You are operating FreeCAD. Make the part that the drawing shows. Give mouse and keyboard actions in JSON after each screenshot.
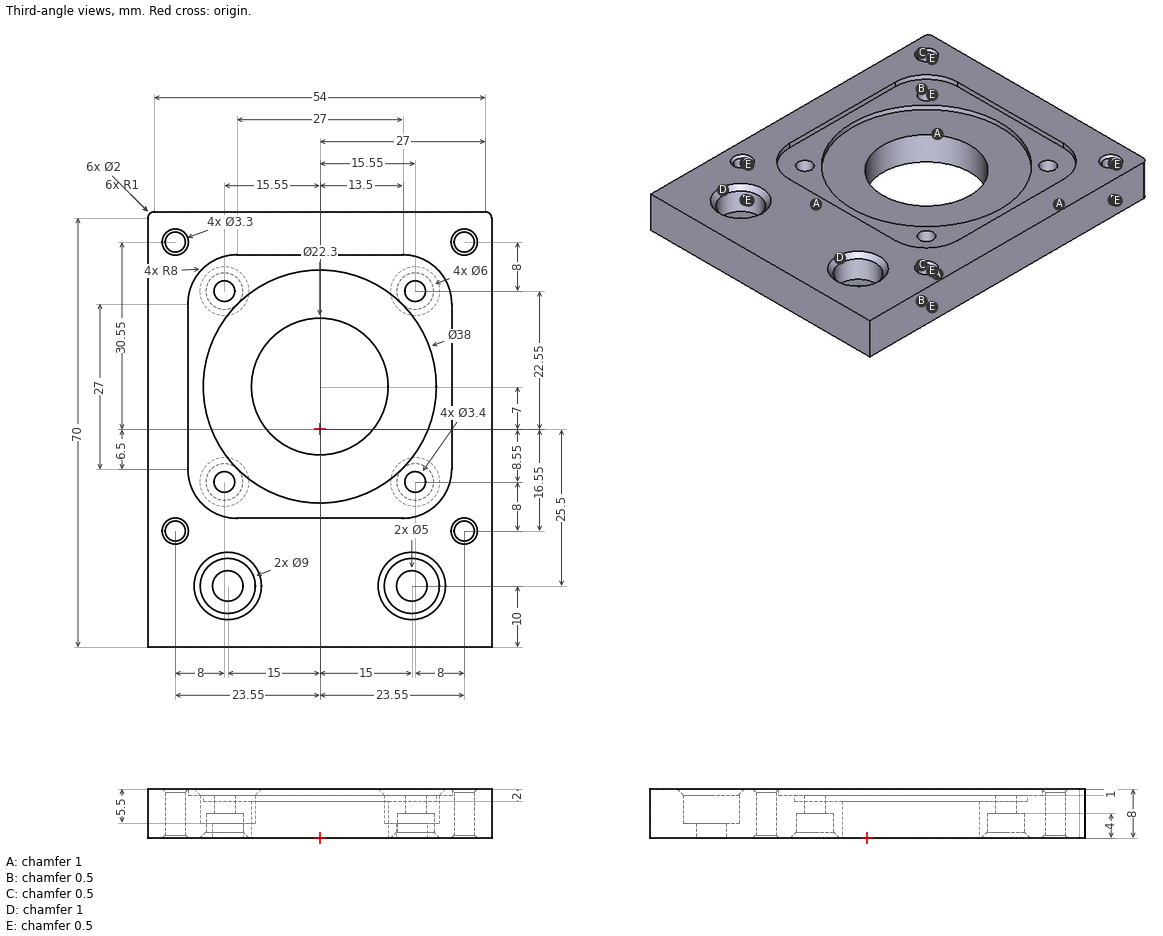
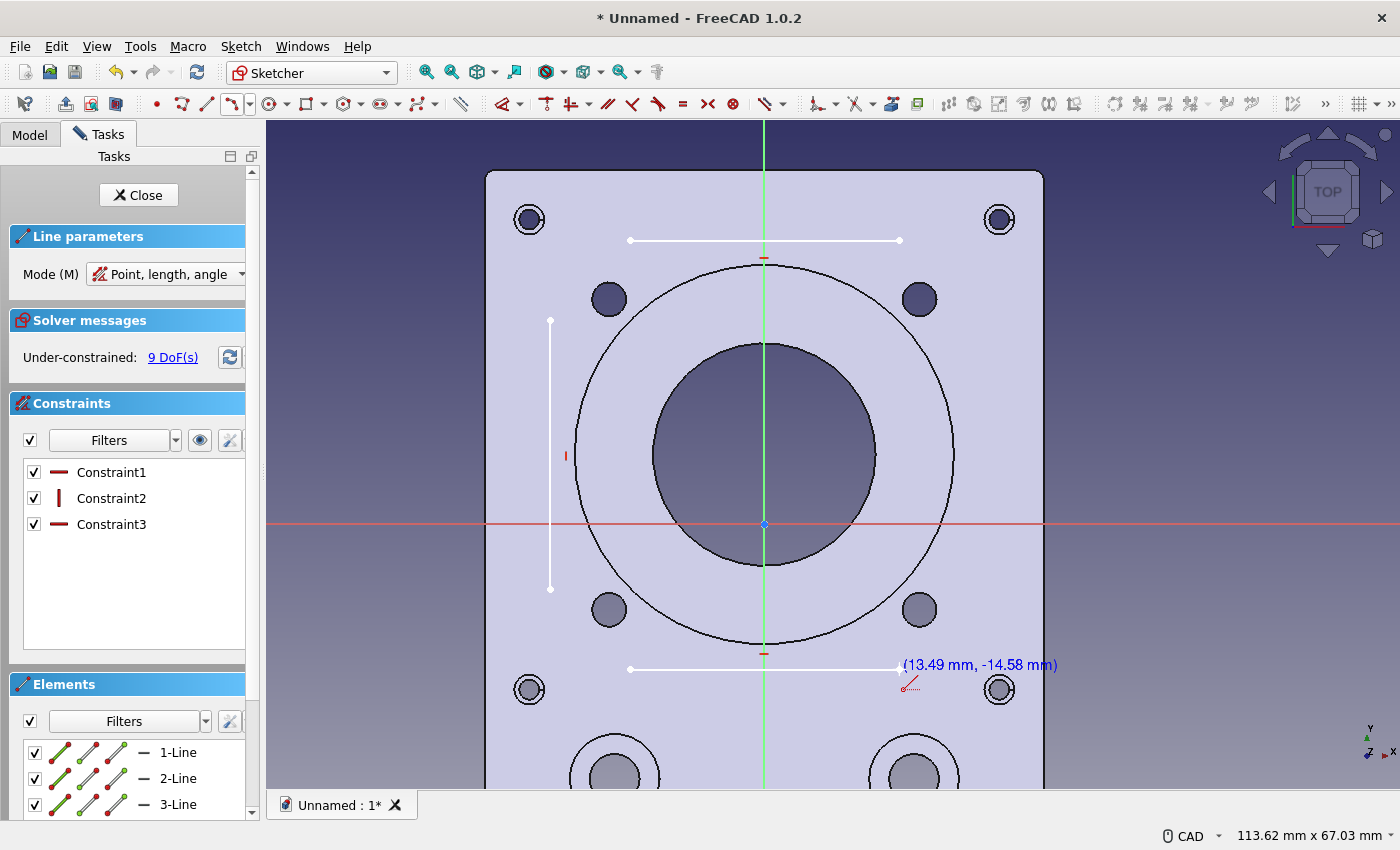
{"action": "left_click", "coordinate": [979, 589]}
{"action": "left_click", "coordinate": [979, 320]}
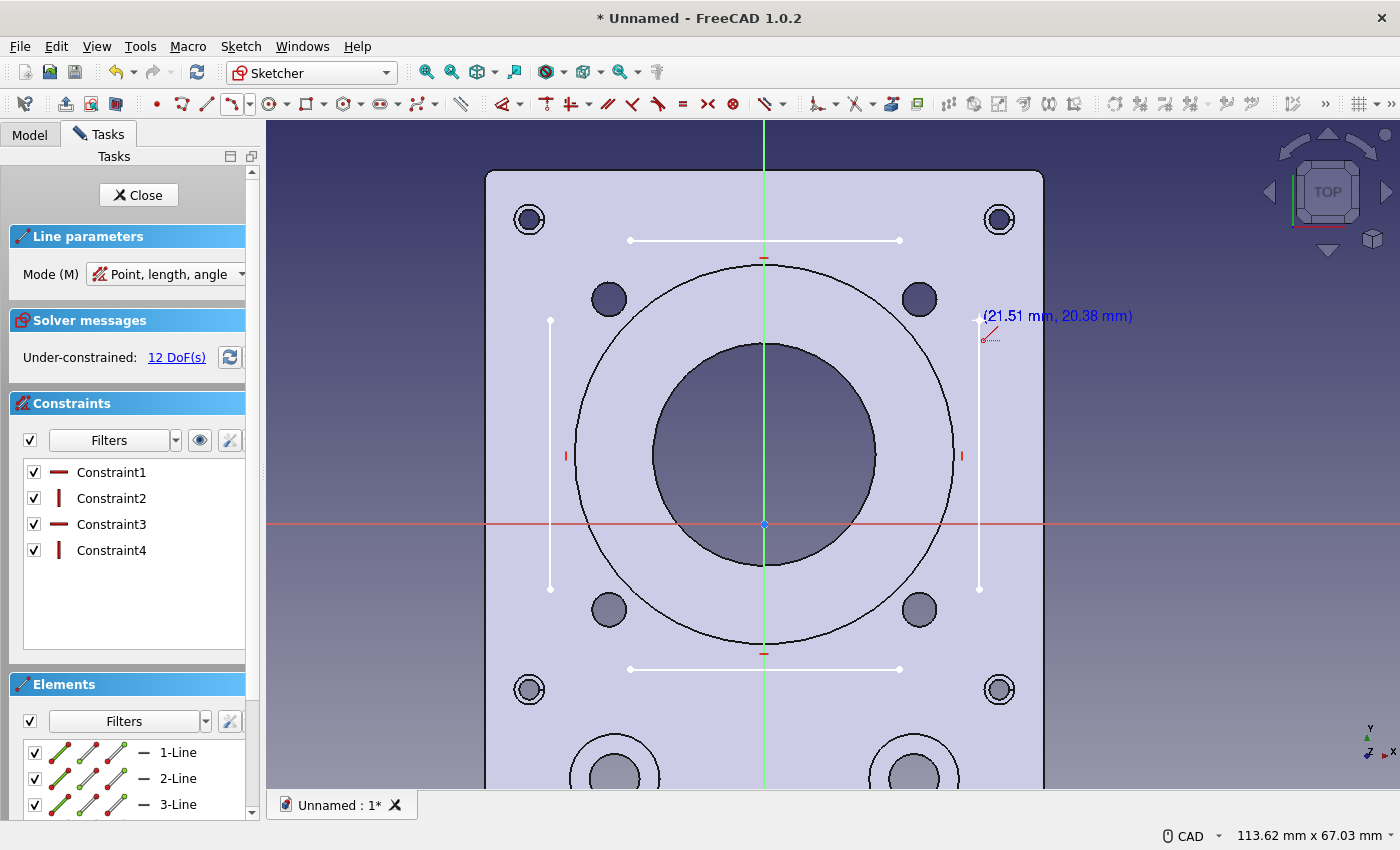
{"action": "key", "text": "g 3 a"}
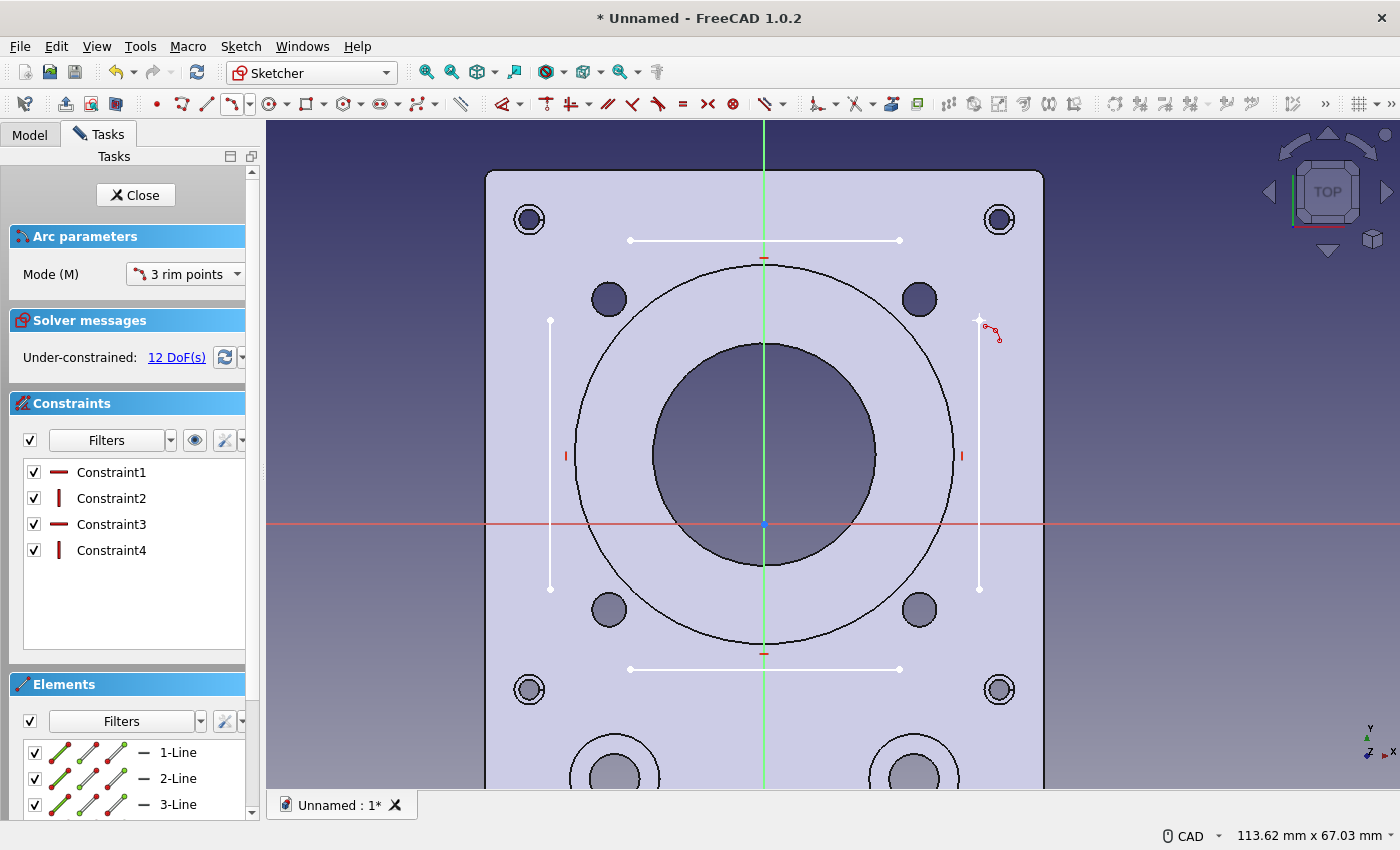
{"action": "left_click", "coordinate": [630, 241]}
{"action": "left_click", "coordinate": [550, 321]}
{"action": "left_click", "coordinate": [573, 263]}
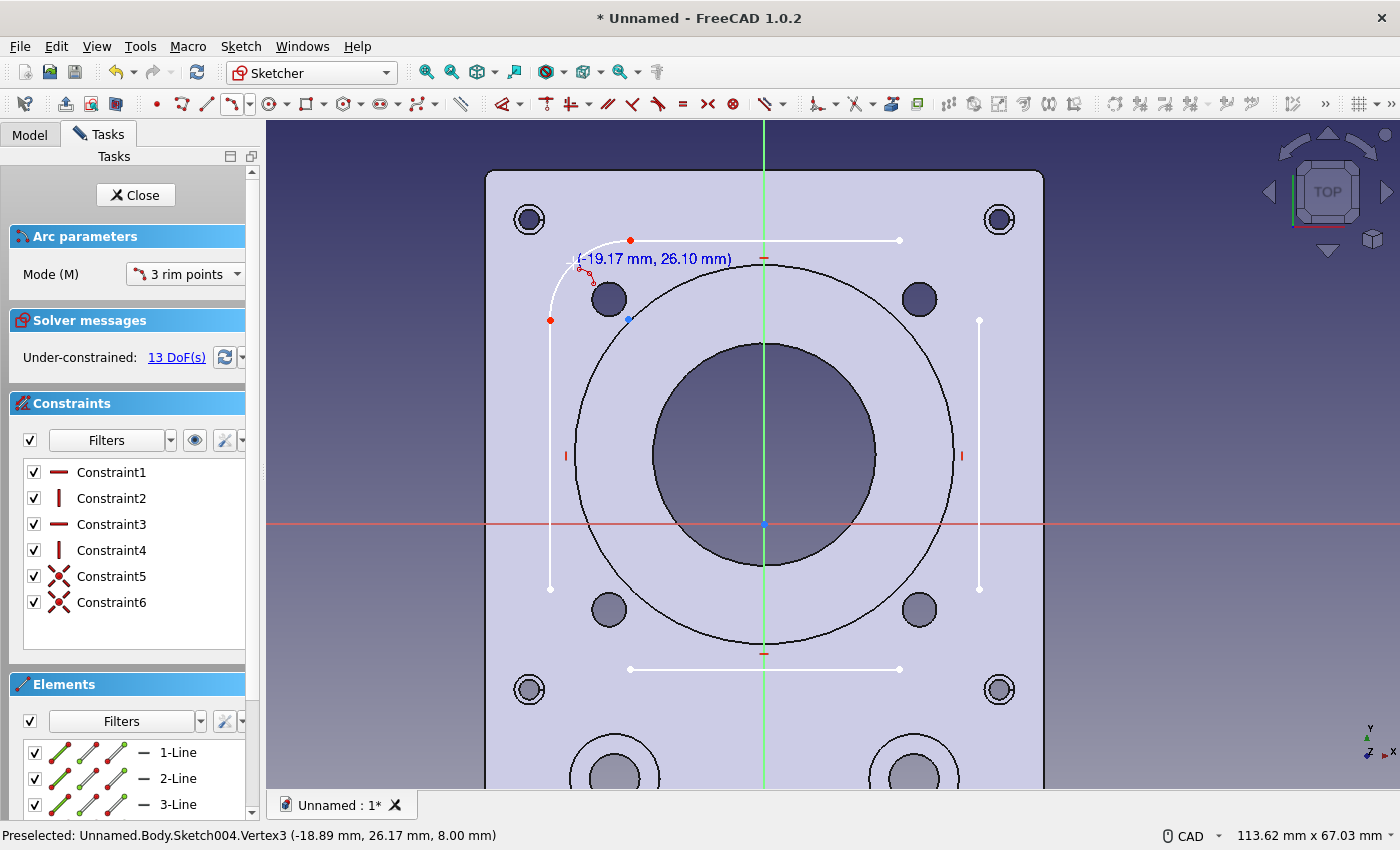
{"action": "left_click", "coordinate": [550, 590]}
{"action": "left_click", "coordinate": [630, 670]}
{"action": "left_click", "coordinate": [573, 646]}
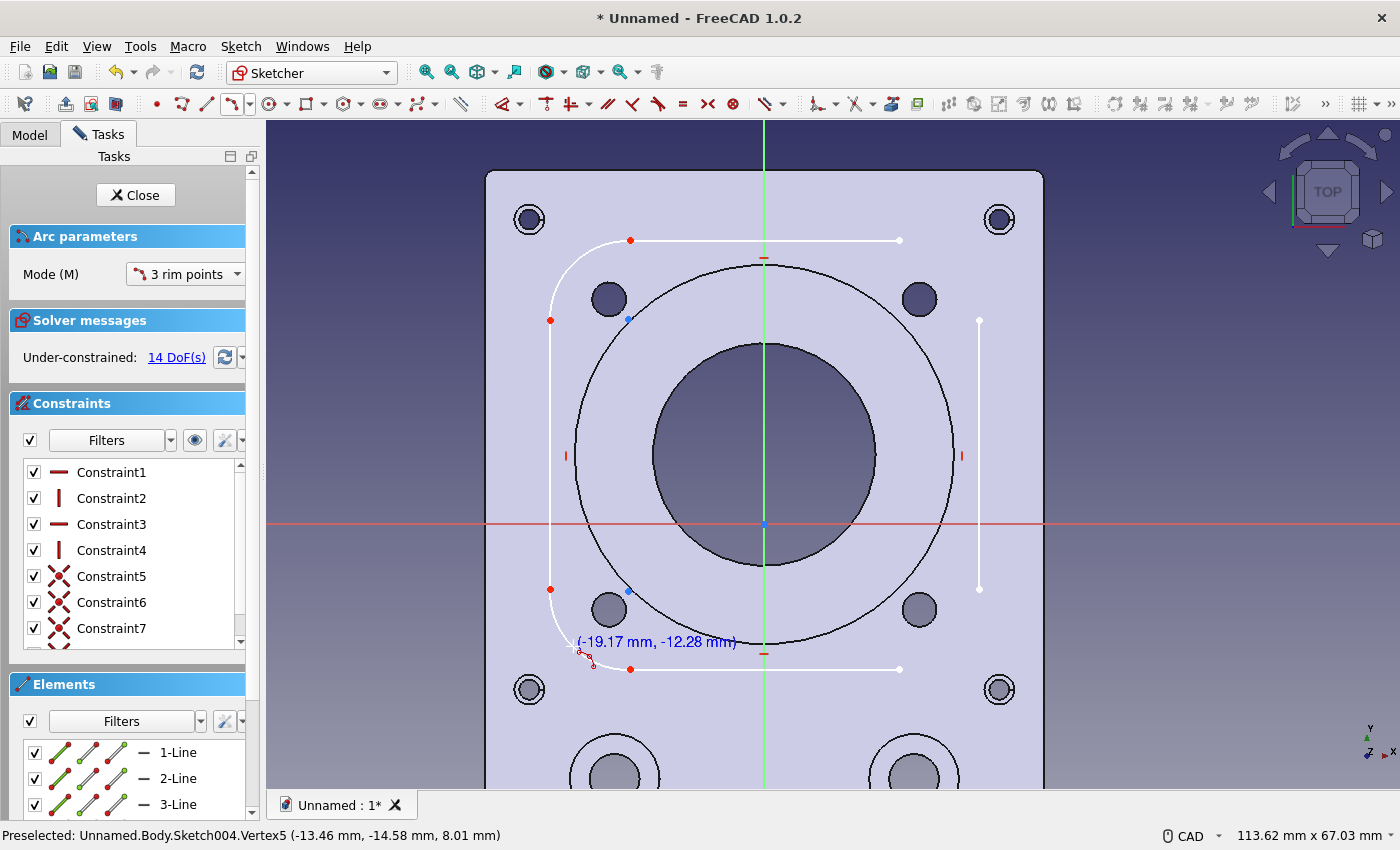
{"action": "left_click", "coordinate": [899, 670]}
{"action": "left_click", "coordinate": [979, 590]}
{"action": "left_click", "coordinate": [956, 646]}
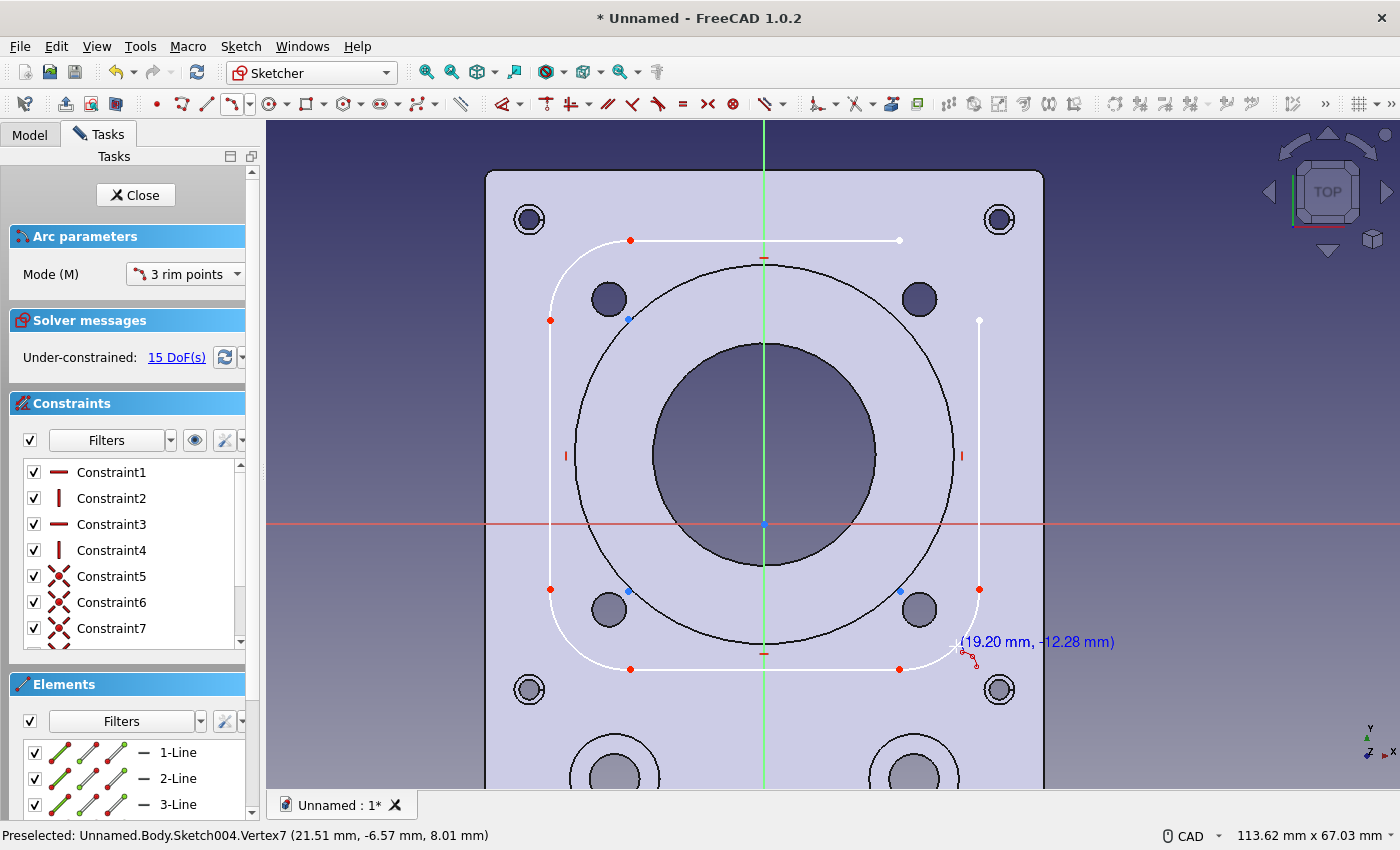
{"action": "left_click", "coordinate": [979, 321]}
{"action": "left_click", "coordinate": [899, 241]}
{"action": "left_click", "coordinate": [956, 263]}
{"action": "key", "text": "Escape"}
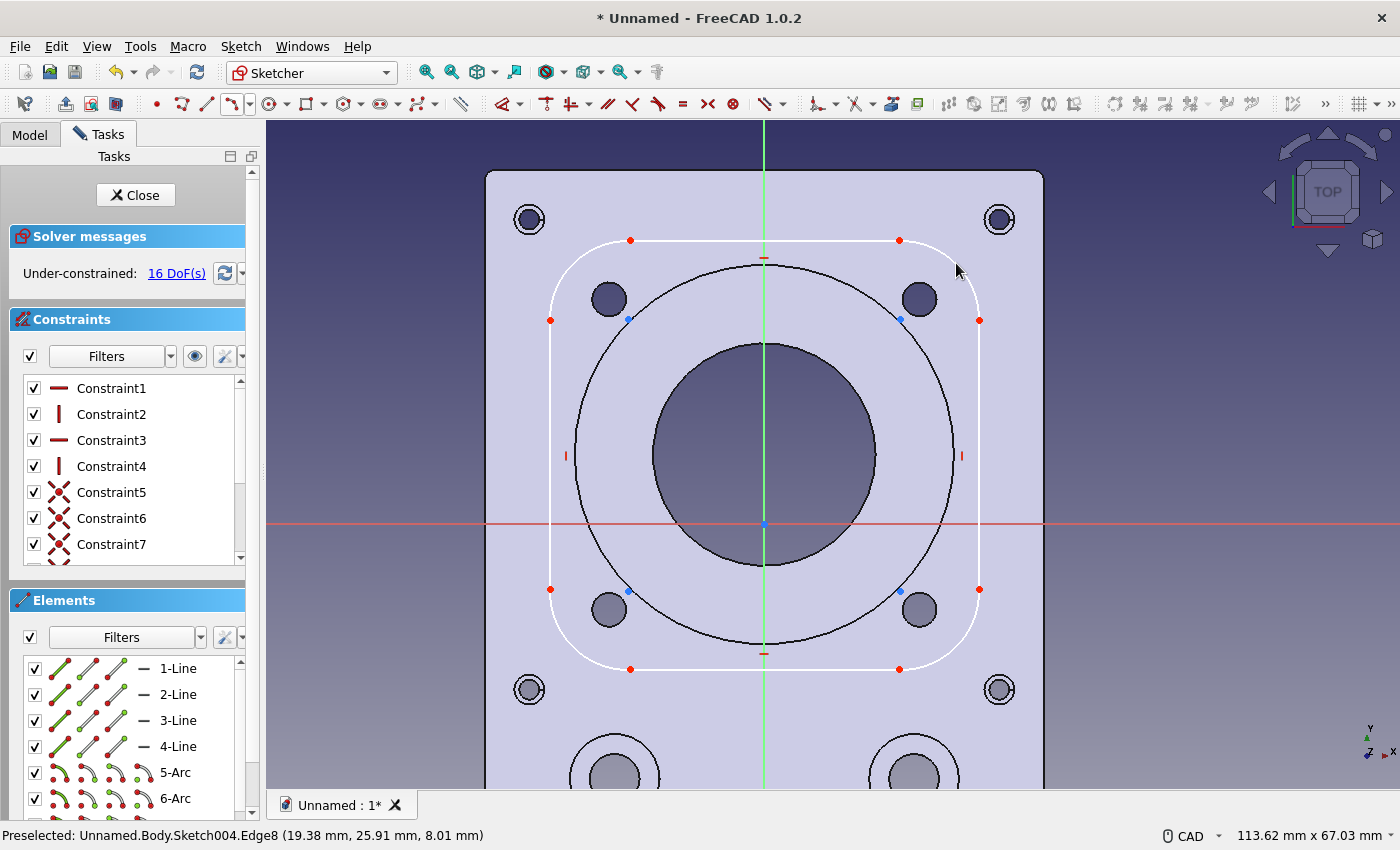
{"action": "left_click", "coordinate": [818, 241]}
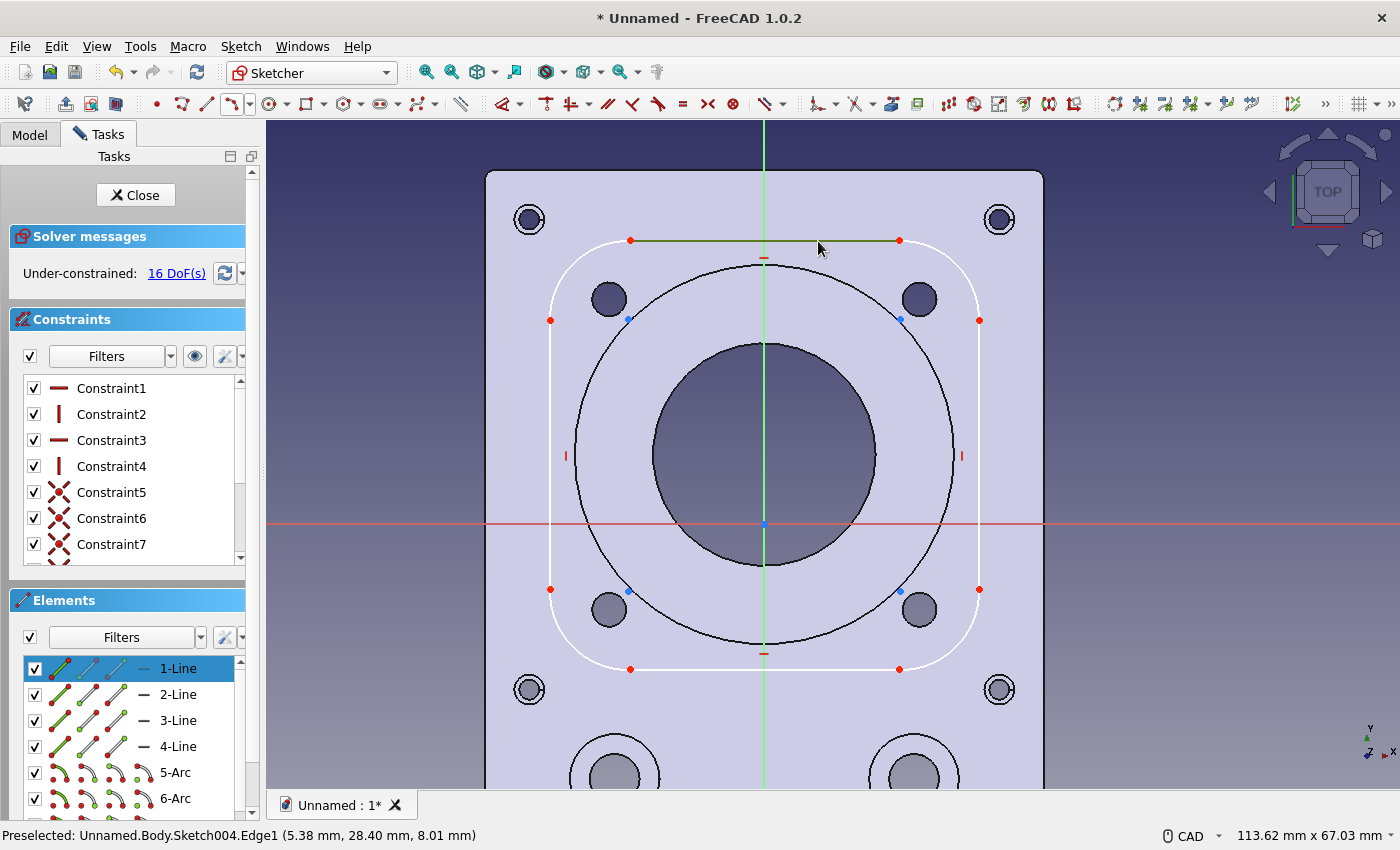
{"action": "left_click", "coordinate": [593, 249]}